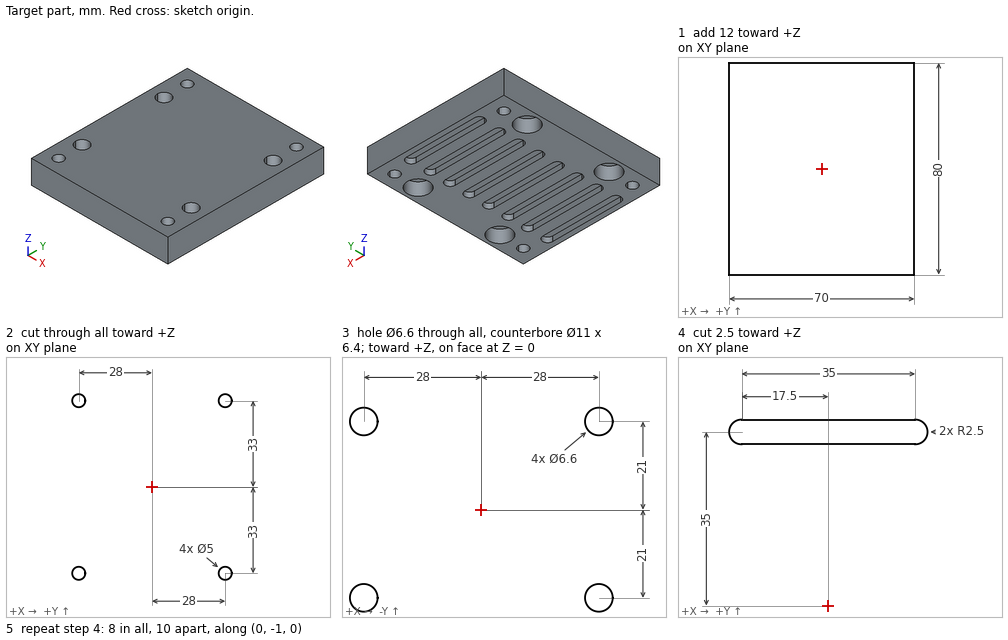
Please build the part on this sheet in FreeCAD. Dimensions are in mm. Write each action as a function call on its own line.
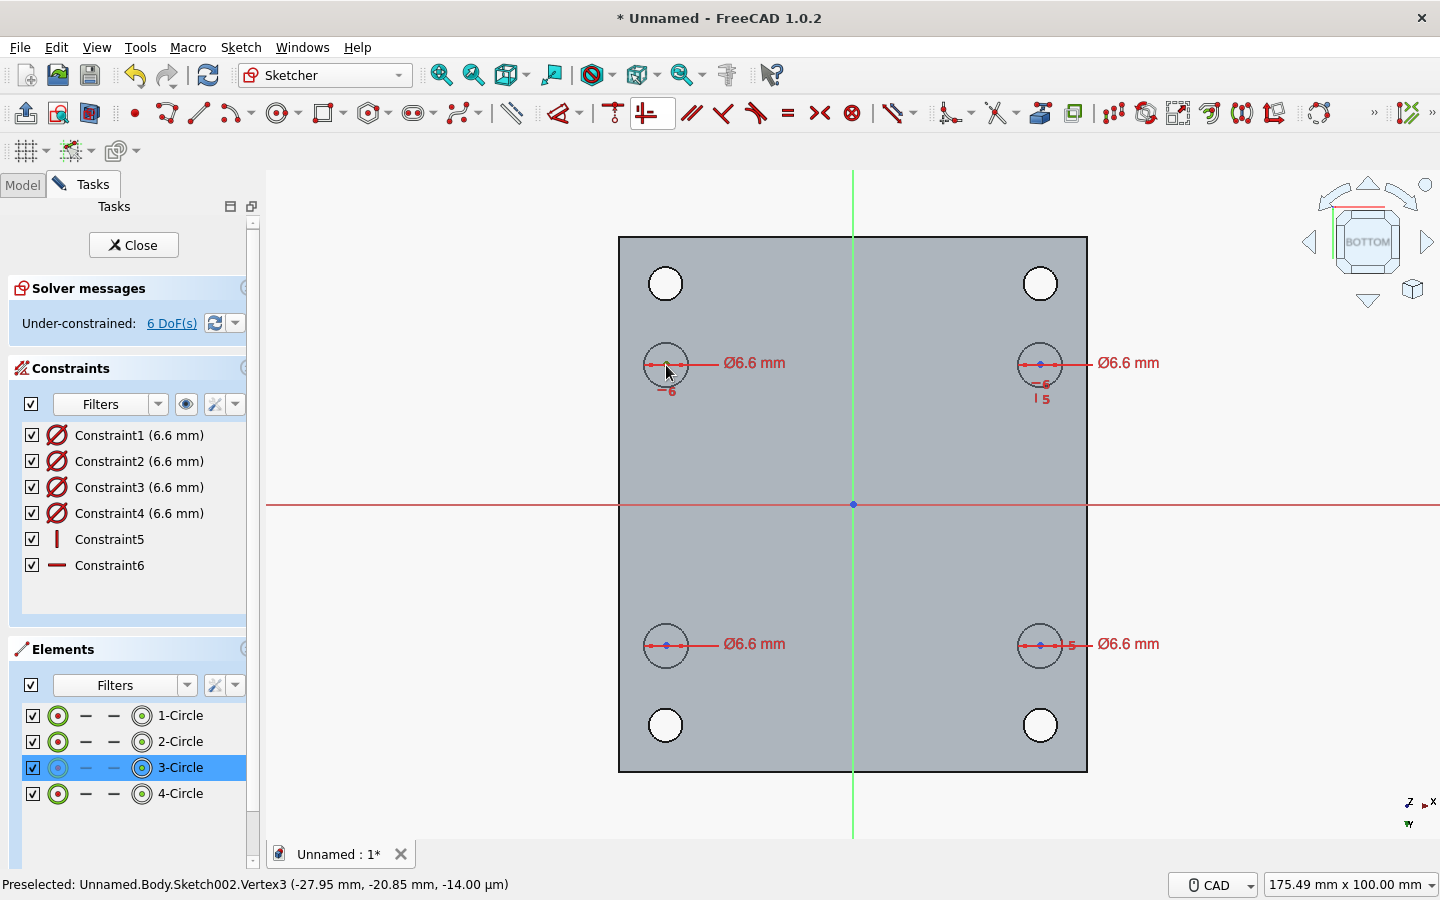
click(666, 646)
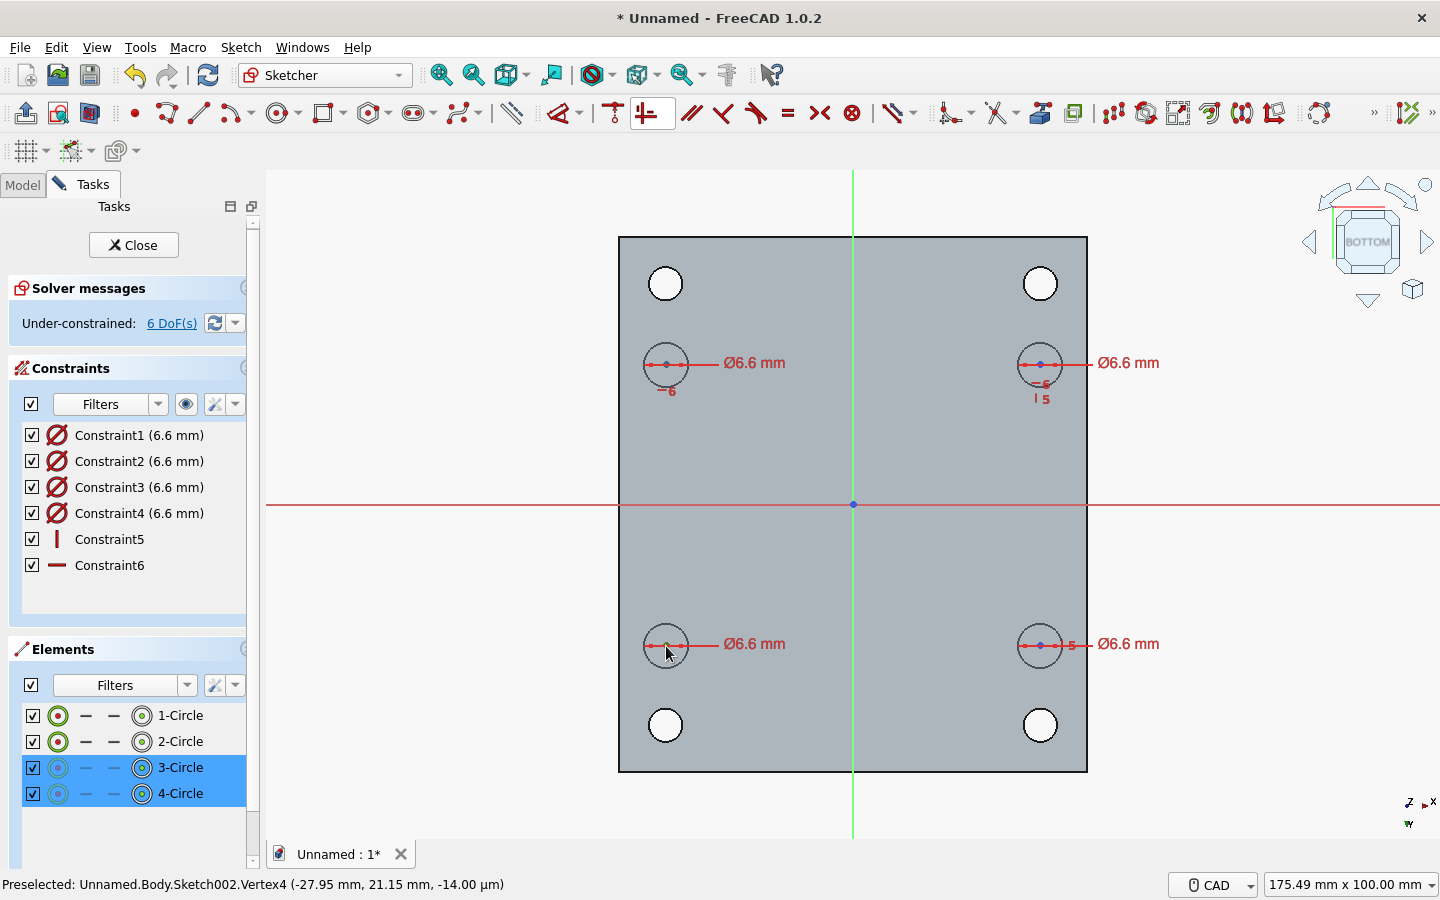
key(v)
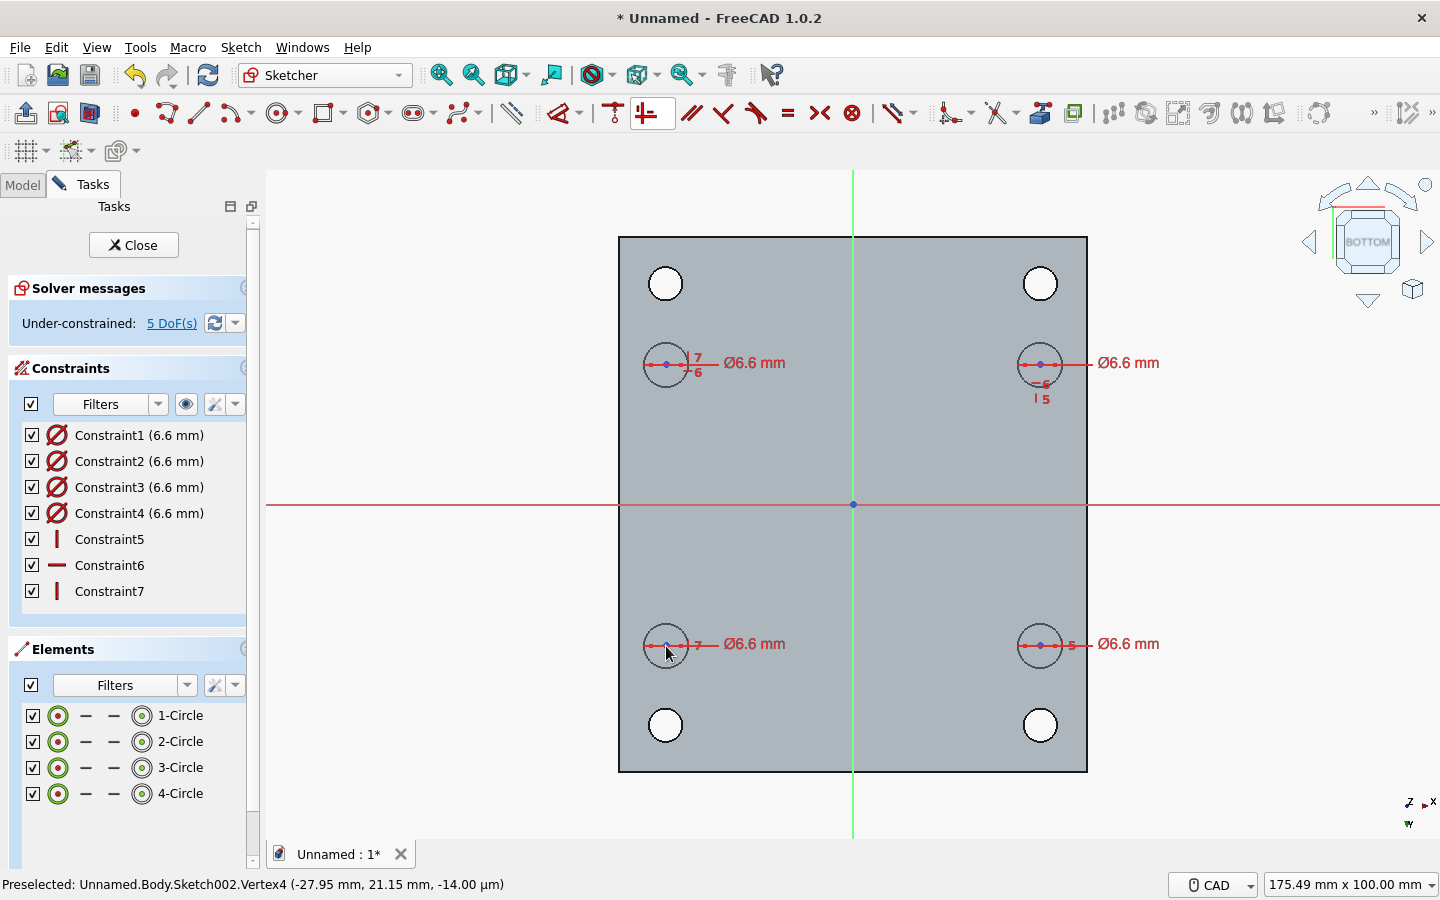
click(1040, 646)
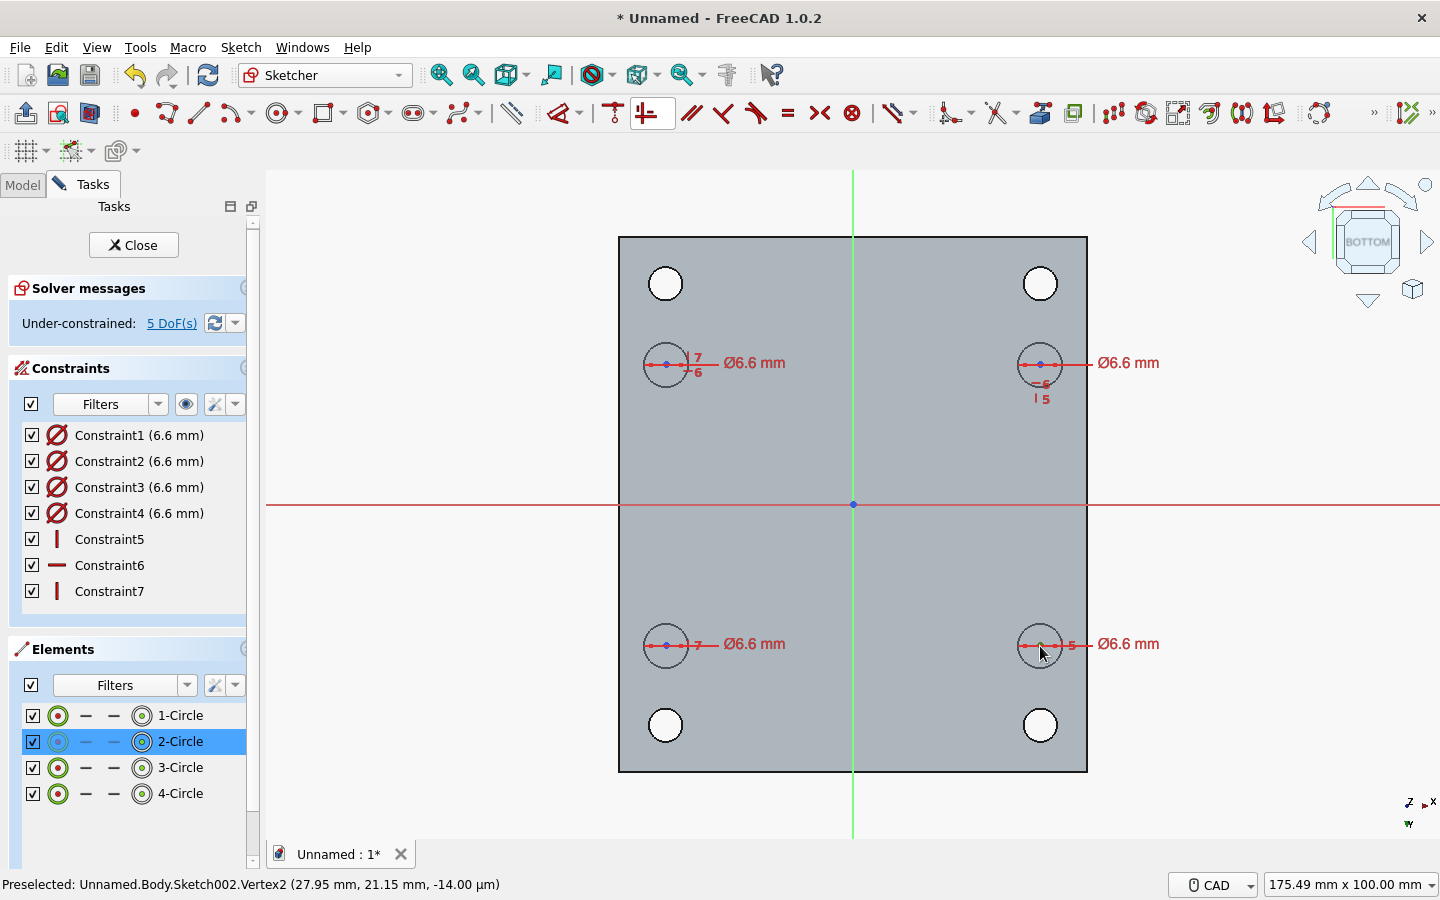
click(666, 646)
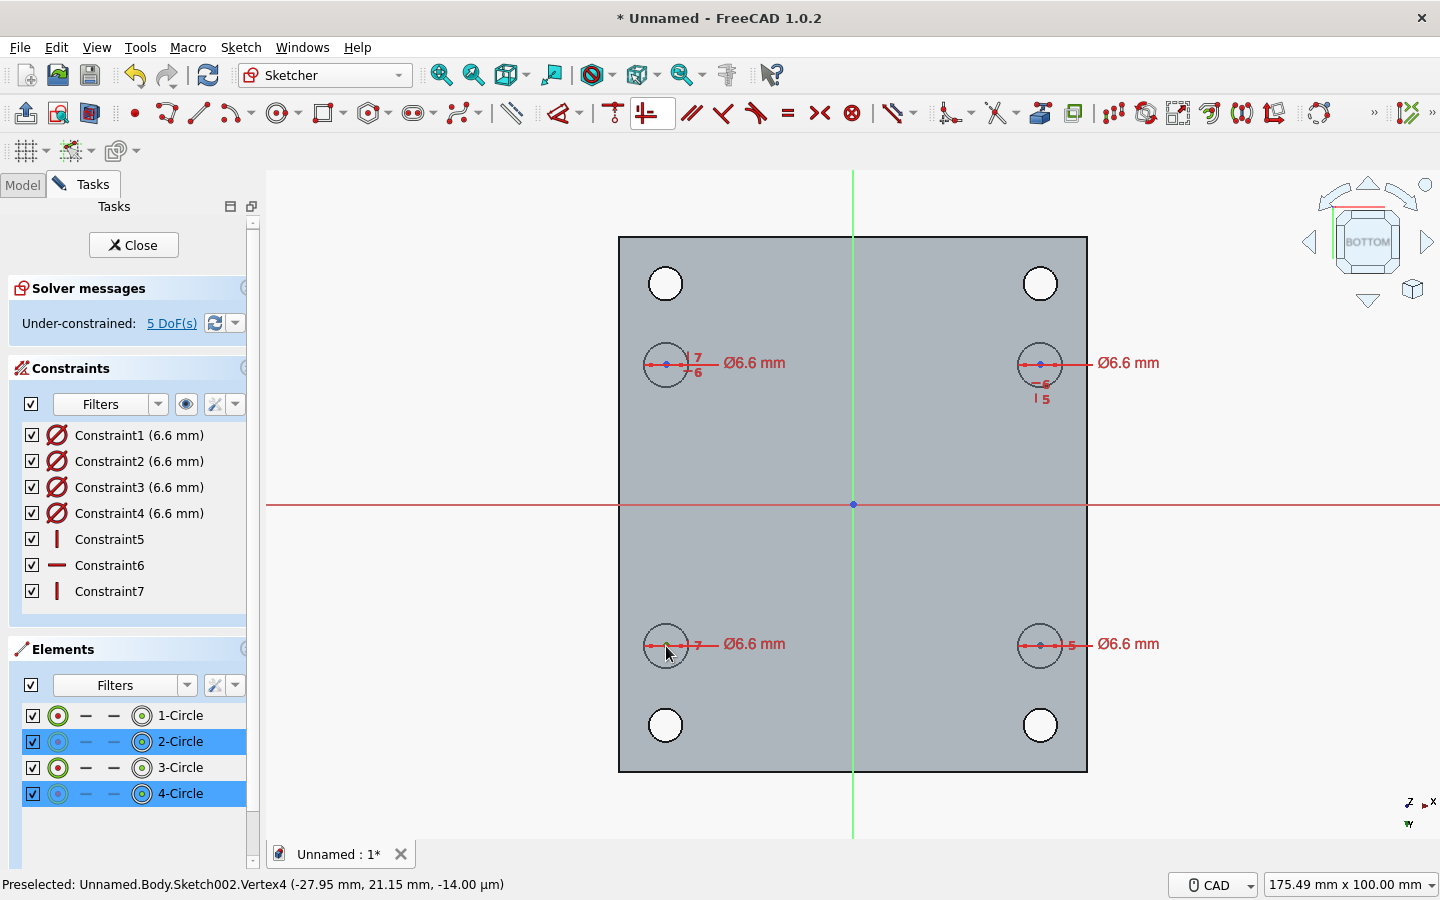
key(h)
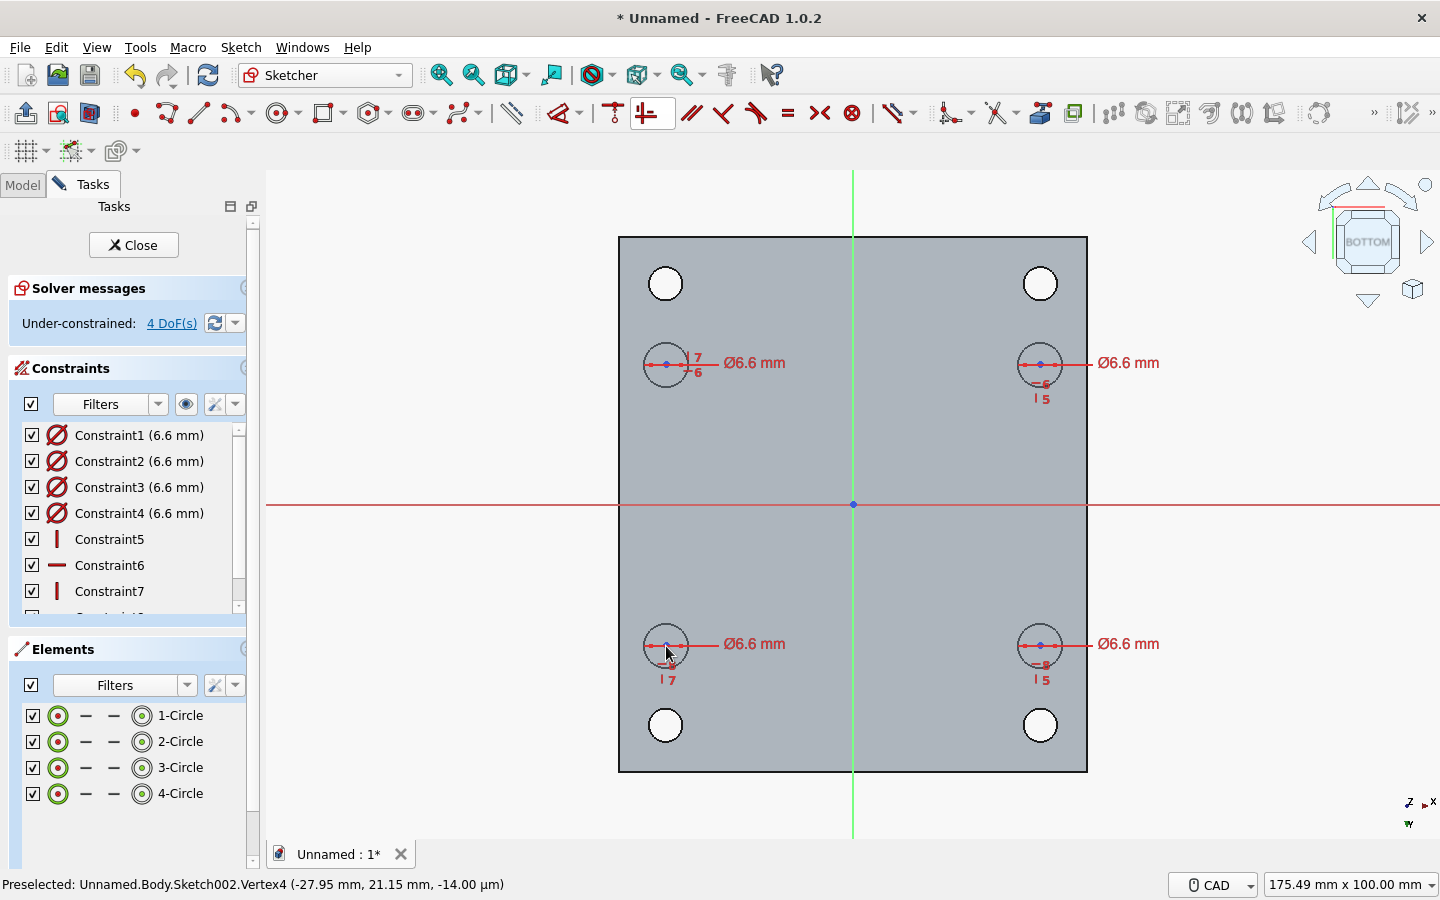
click(558, 114)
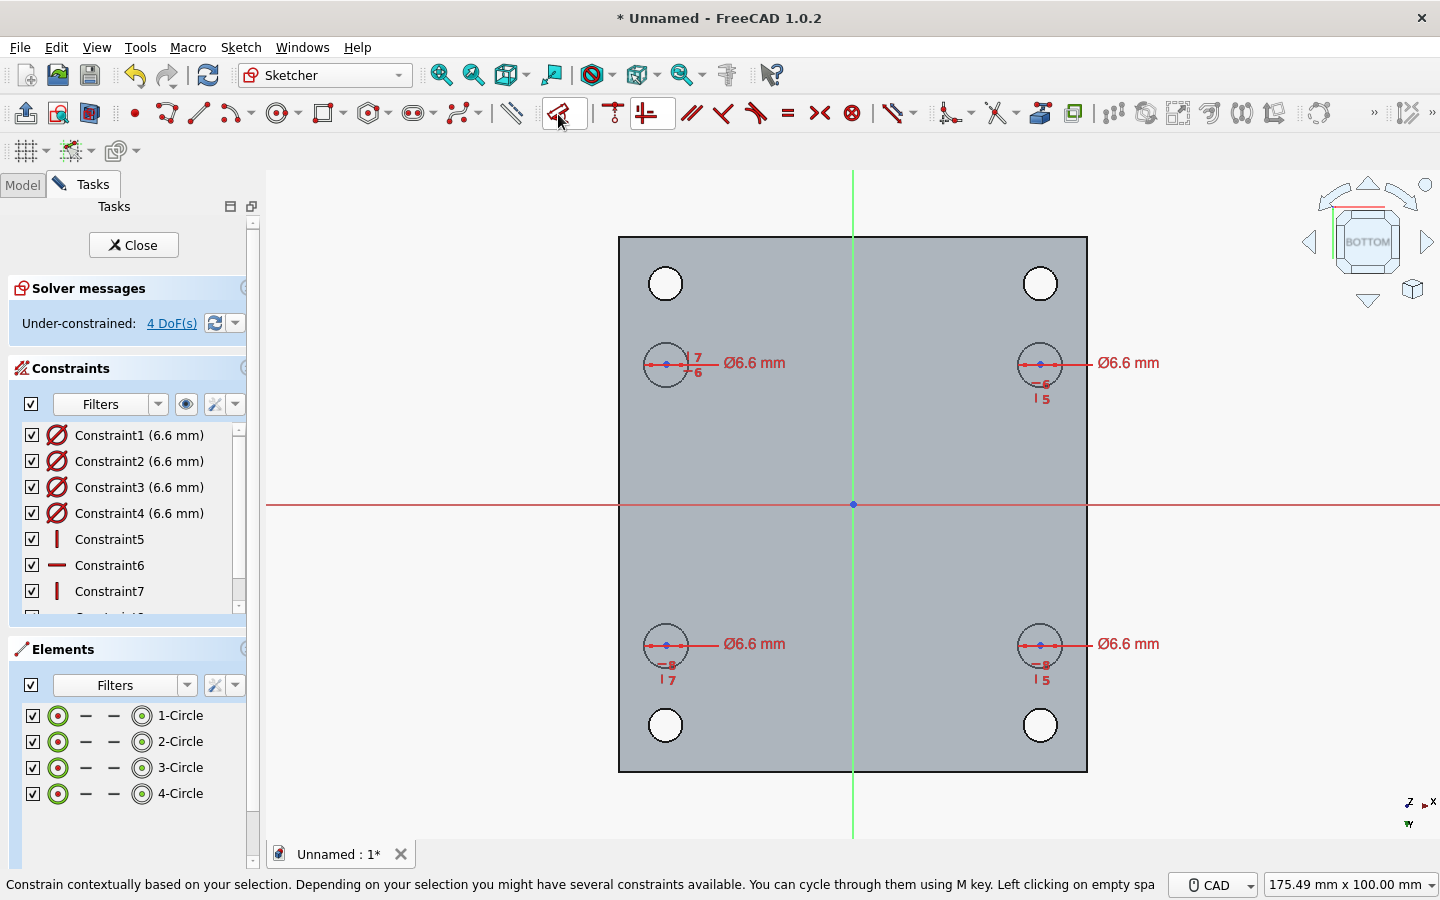
click(1040, 365)
click(946, 331)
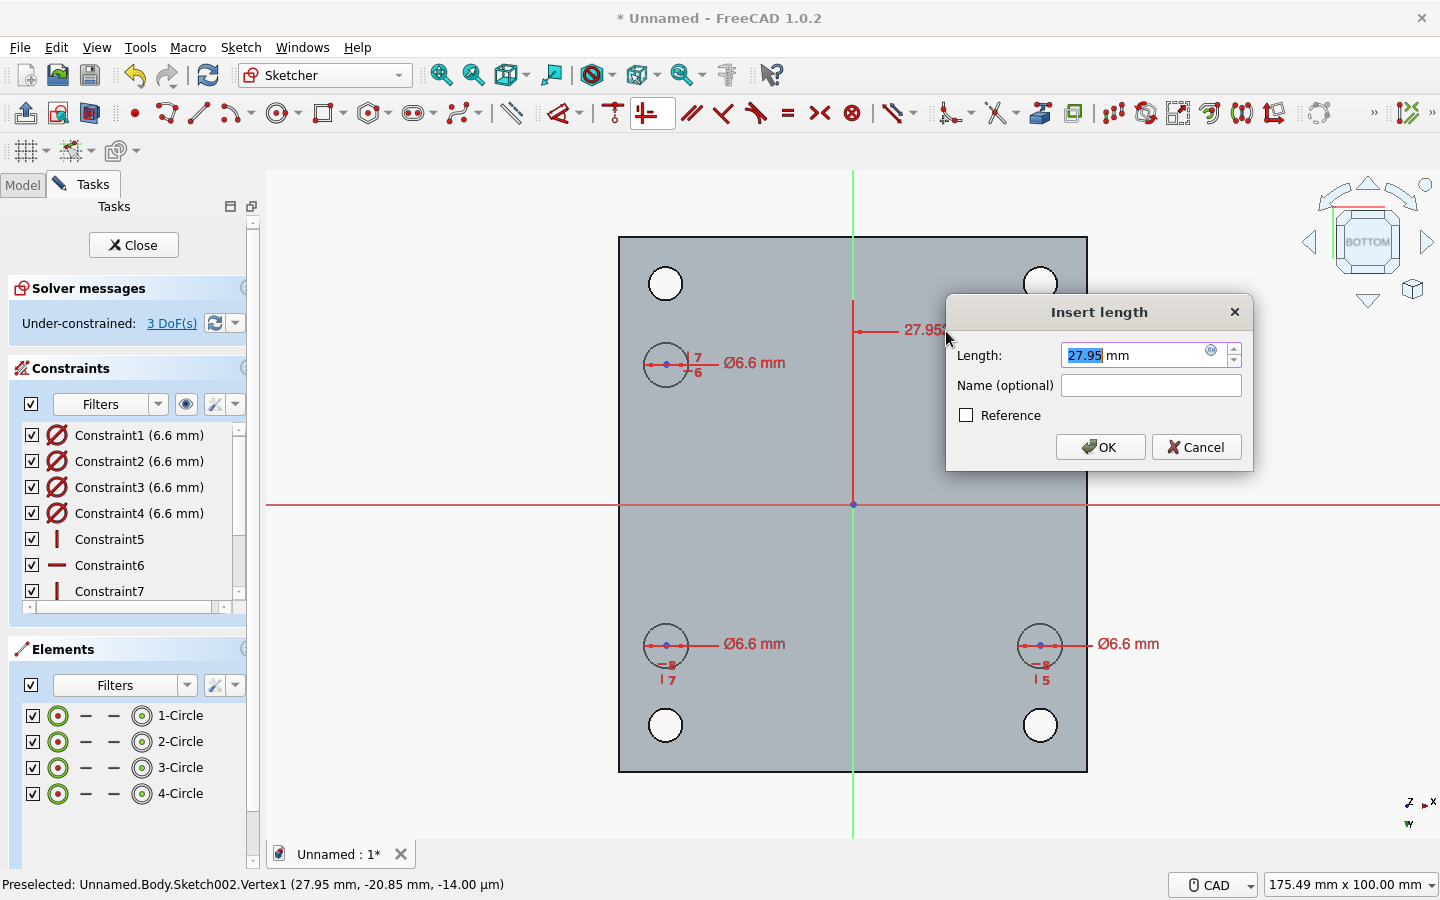
text(28)
key(Return)